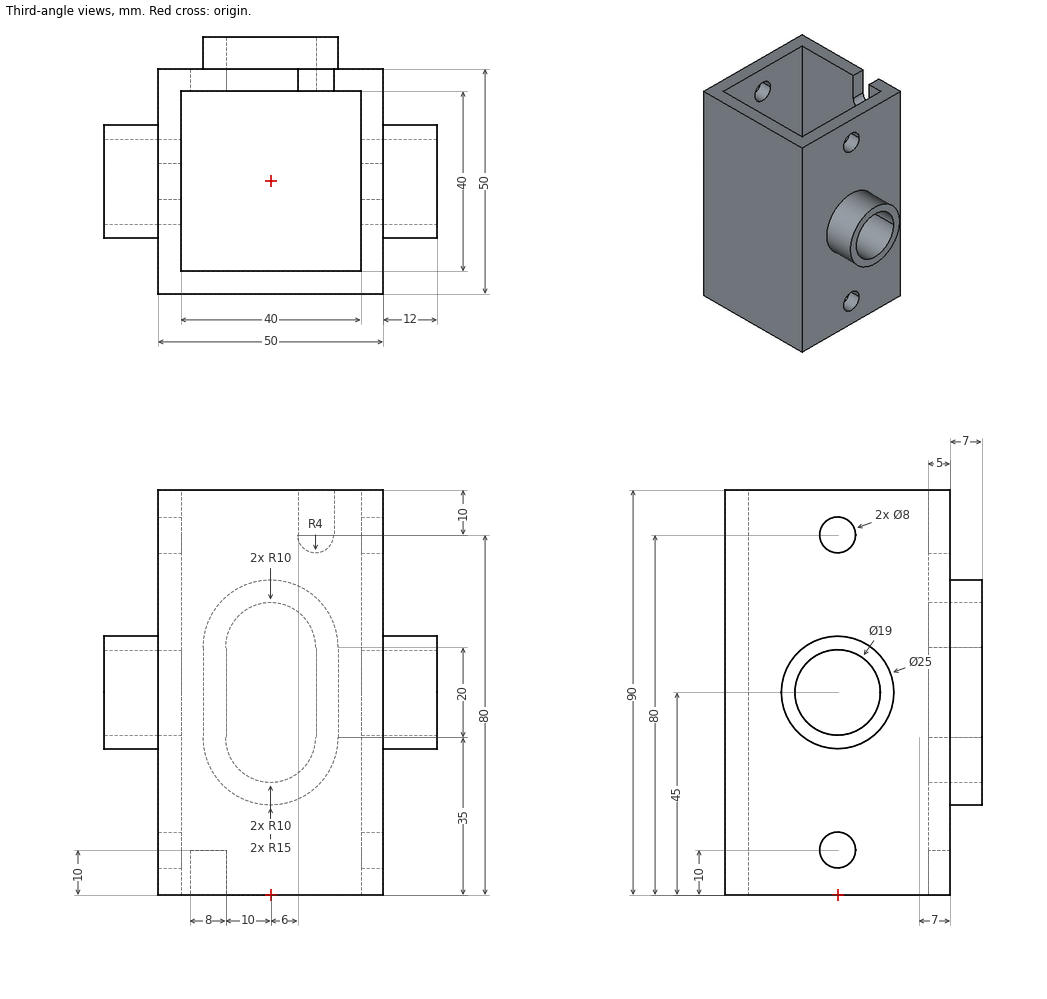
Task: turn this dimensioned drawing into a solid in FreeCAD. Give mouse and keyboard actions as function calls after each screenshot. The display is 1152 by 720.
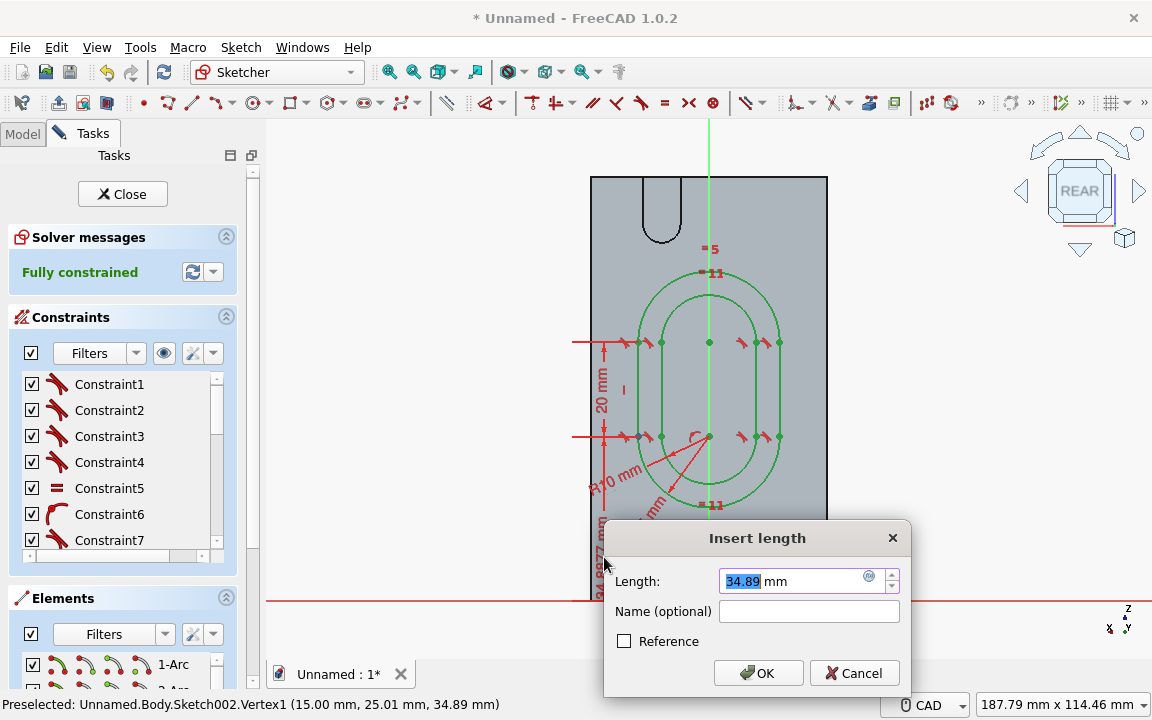
text(35)
key(Return)
key(Escape)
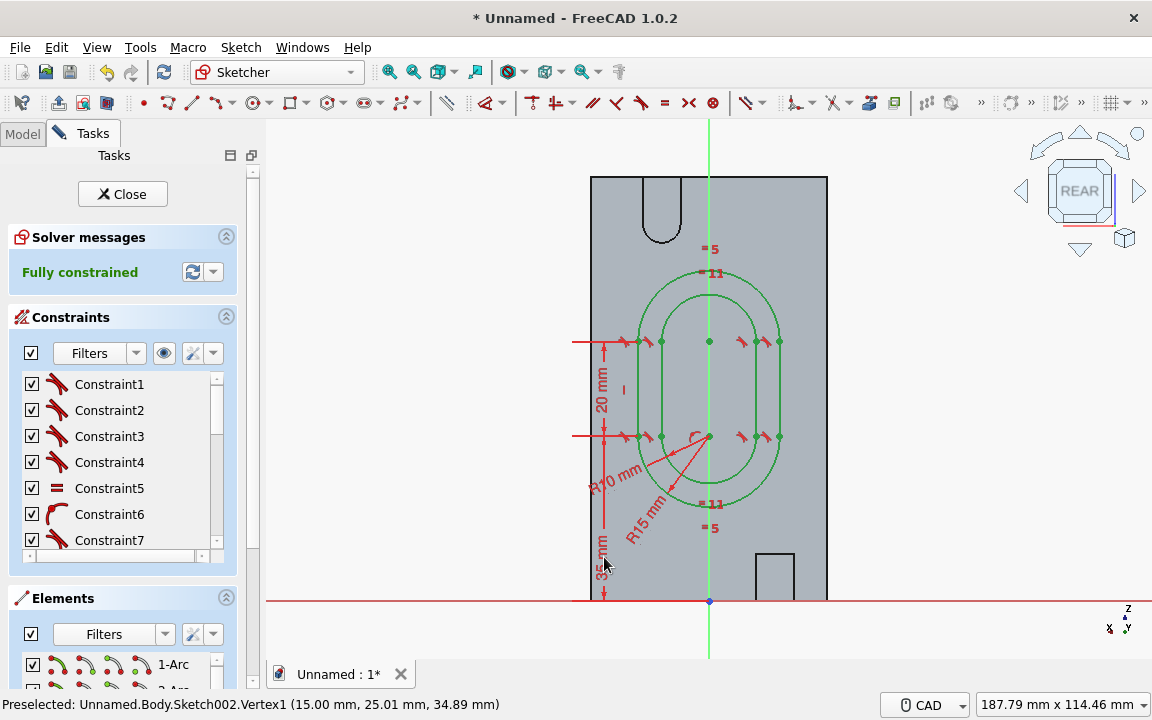
click(123, 194)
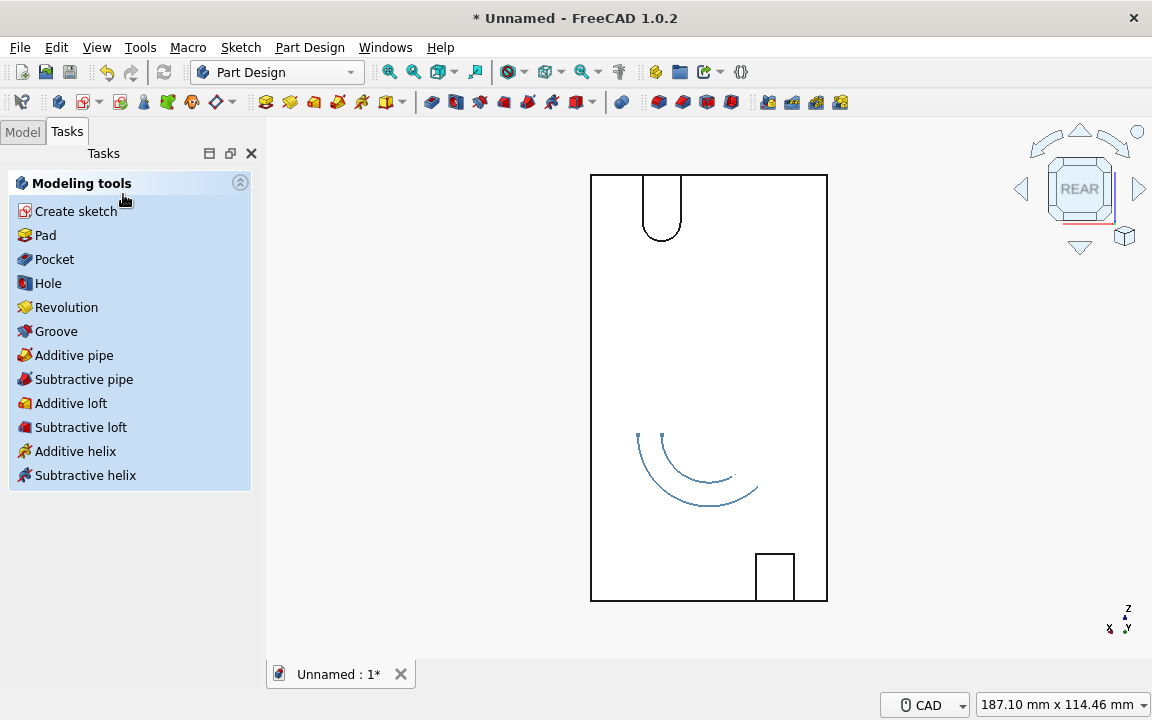
click(266, 102)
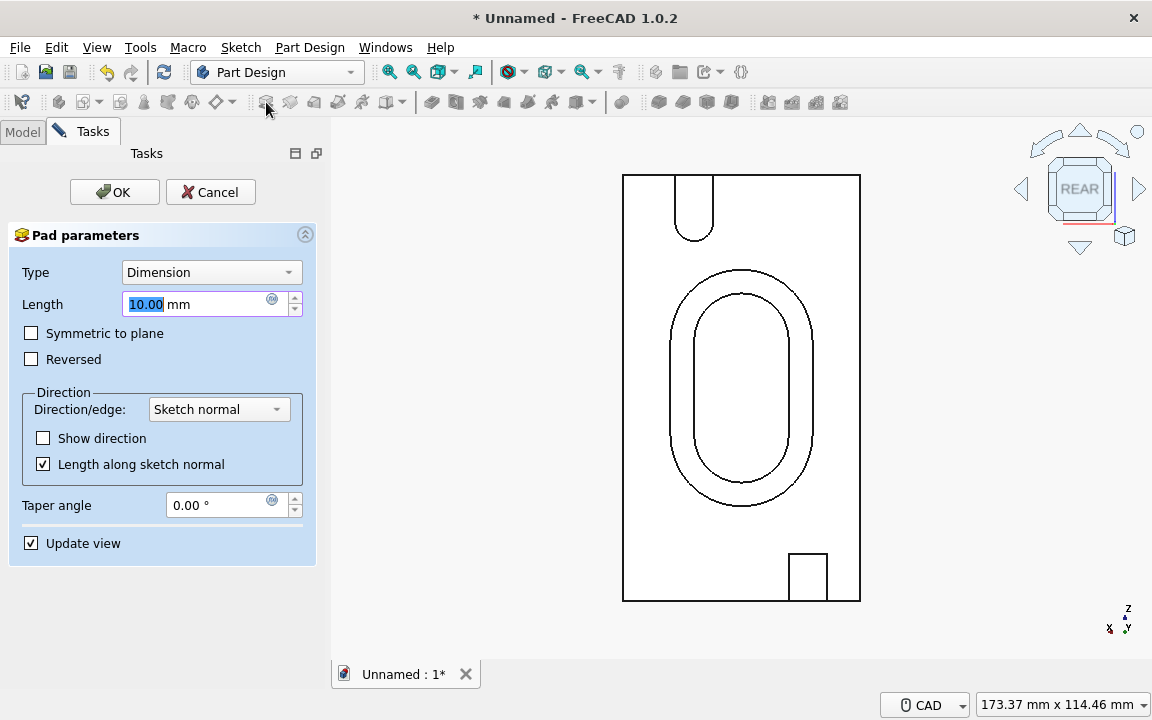
text(7)
key(Tab)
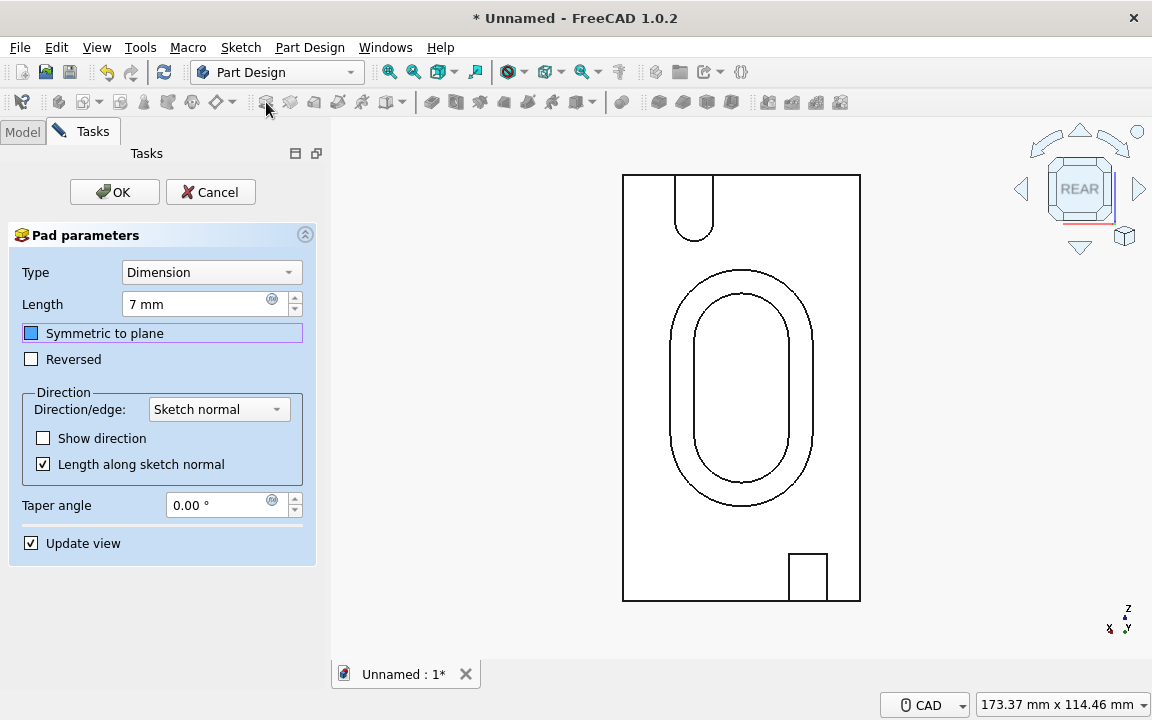
click(115, 192)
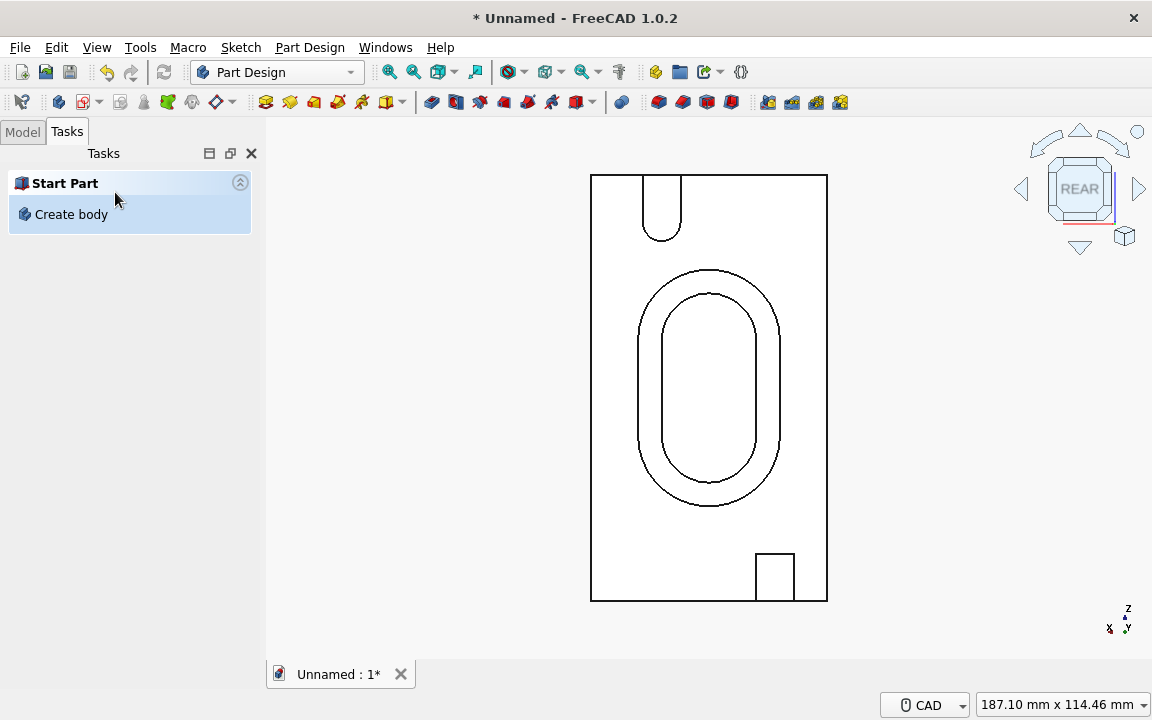
click(23, 131)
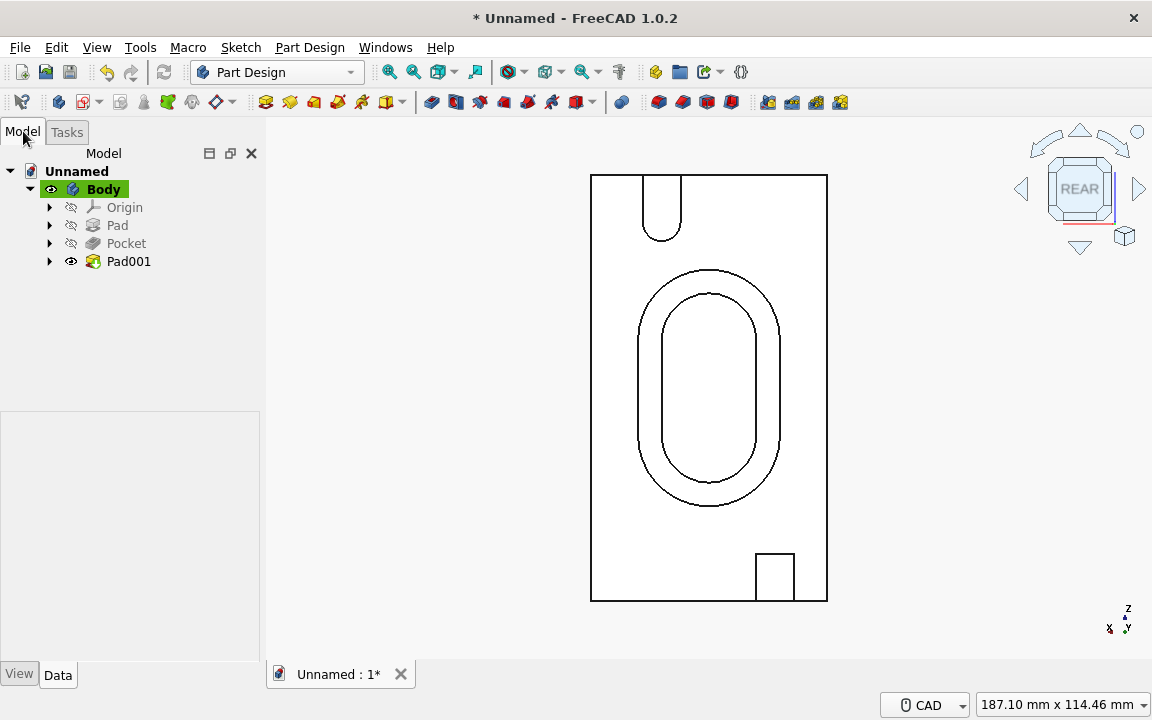
click(50, 207)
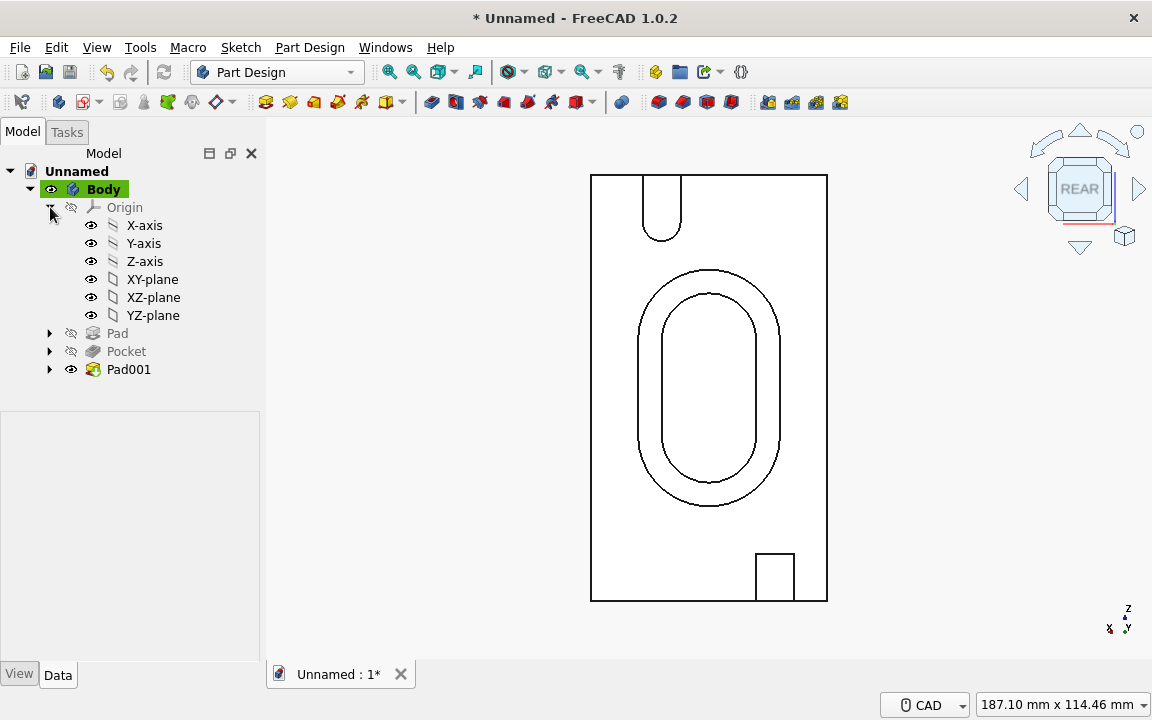
click(136, 297)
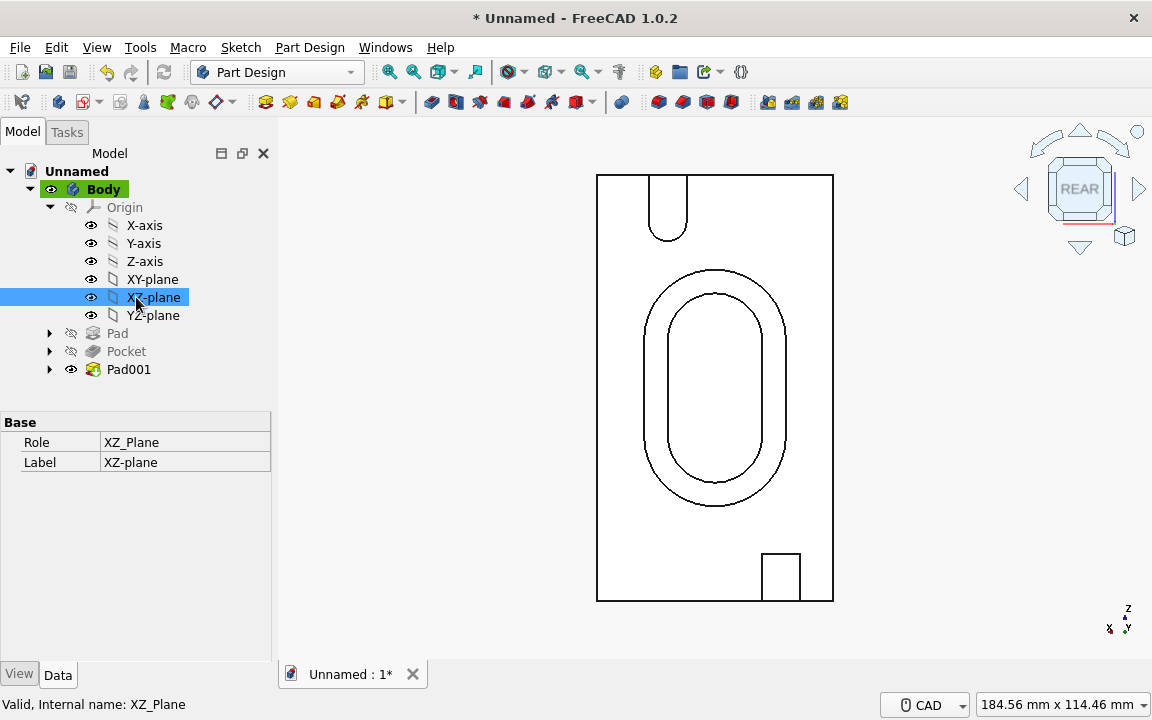
click(216, 102)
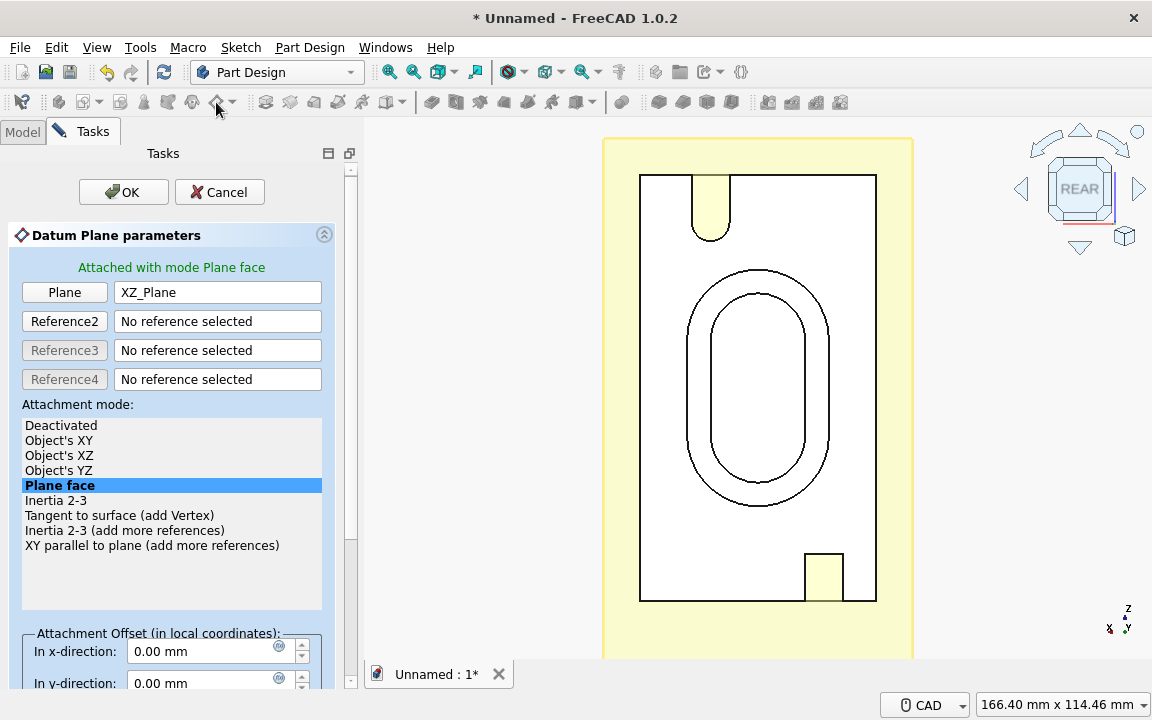
scroll(351, 426, down, 2)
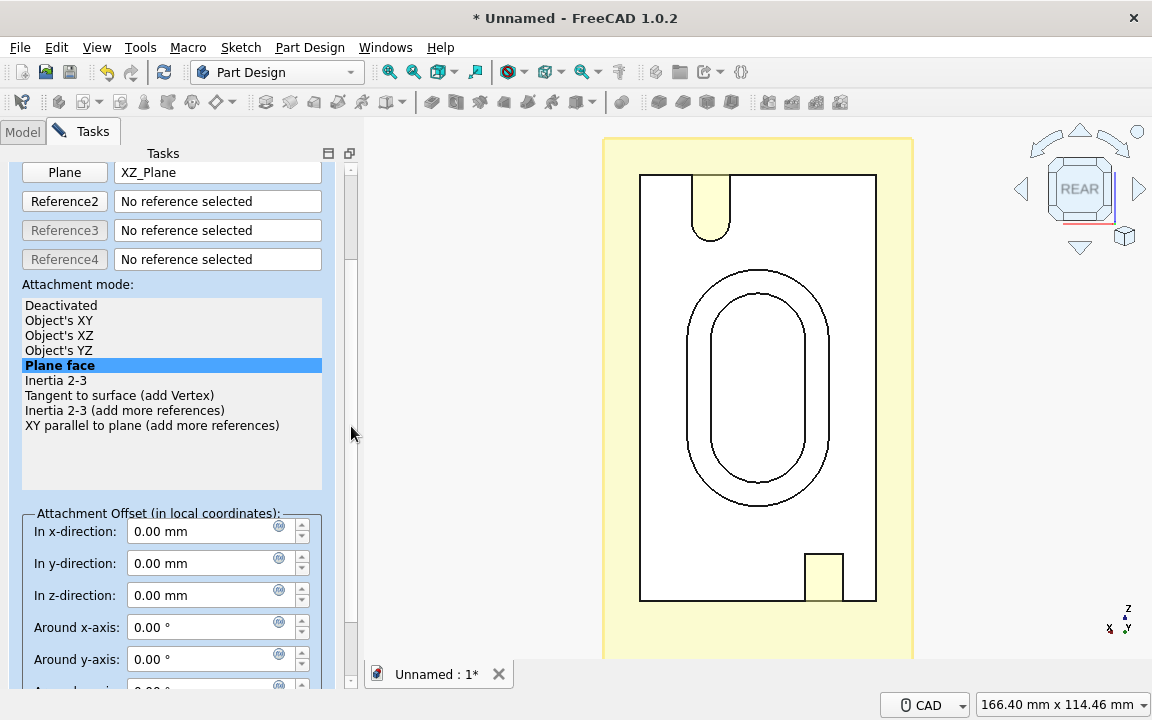
triple_click(210, 595)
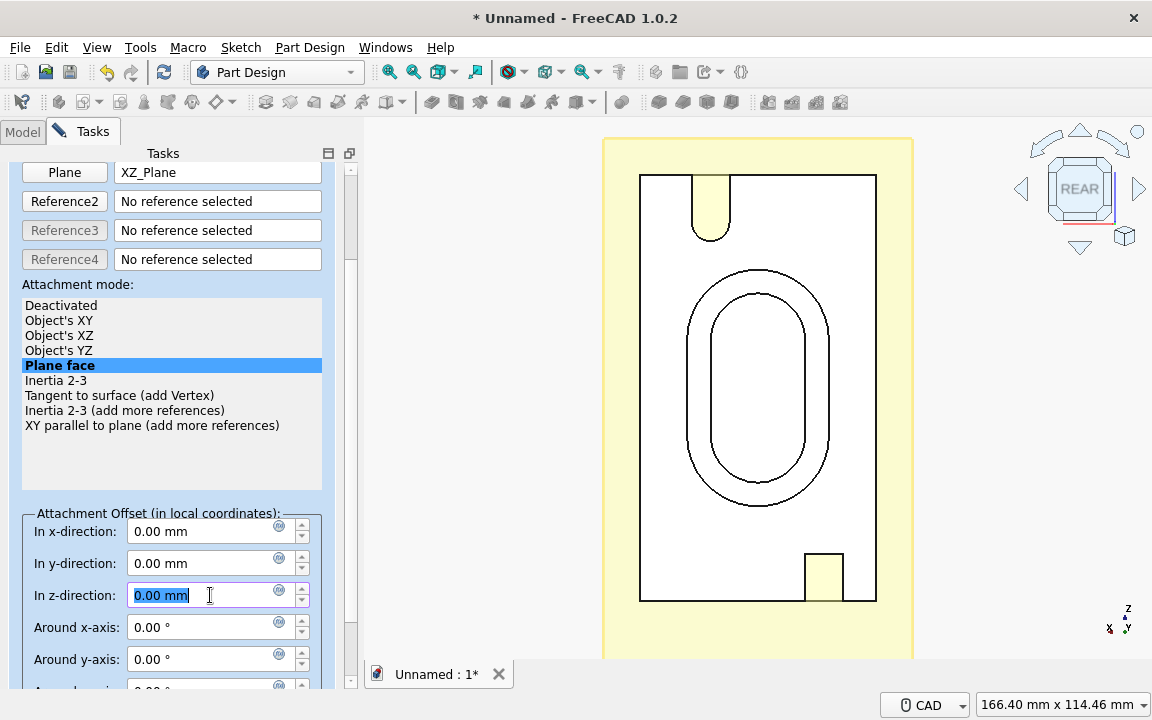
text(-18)
key(Tab)